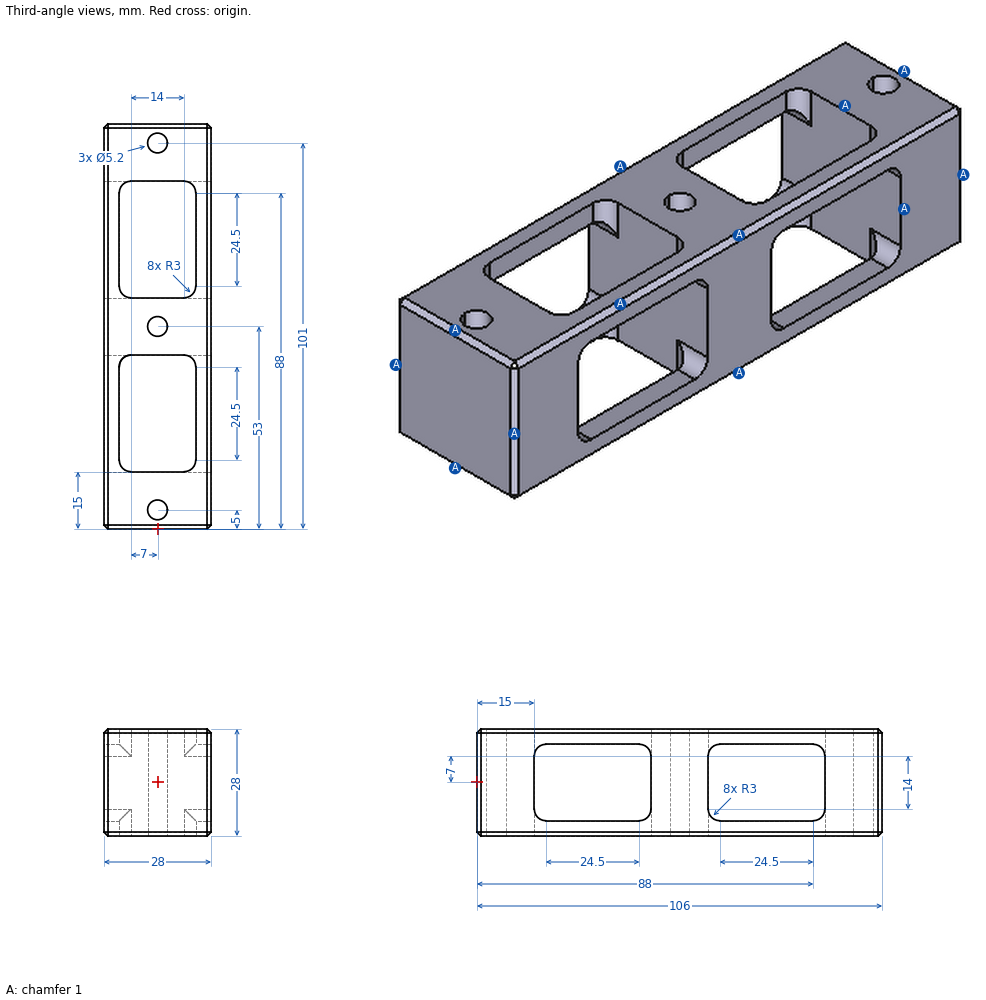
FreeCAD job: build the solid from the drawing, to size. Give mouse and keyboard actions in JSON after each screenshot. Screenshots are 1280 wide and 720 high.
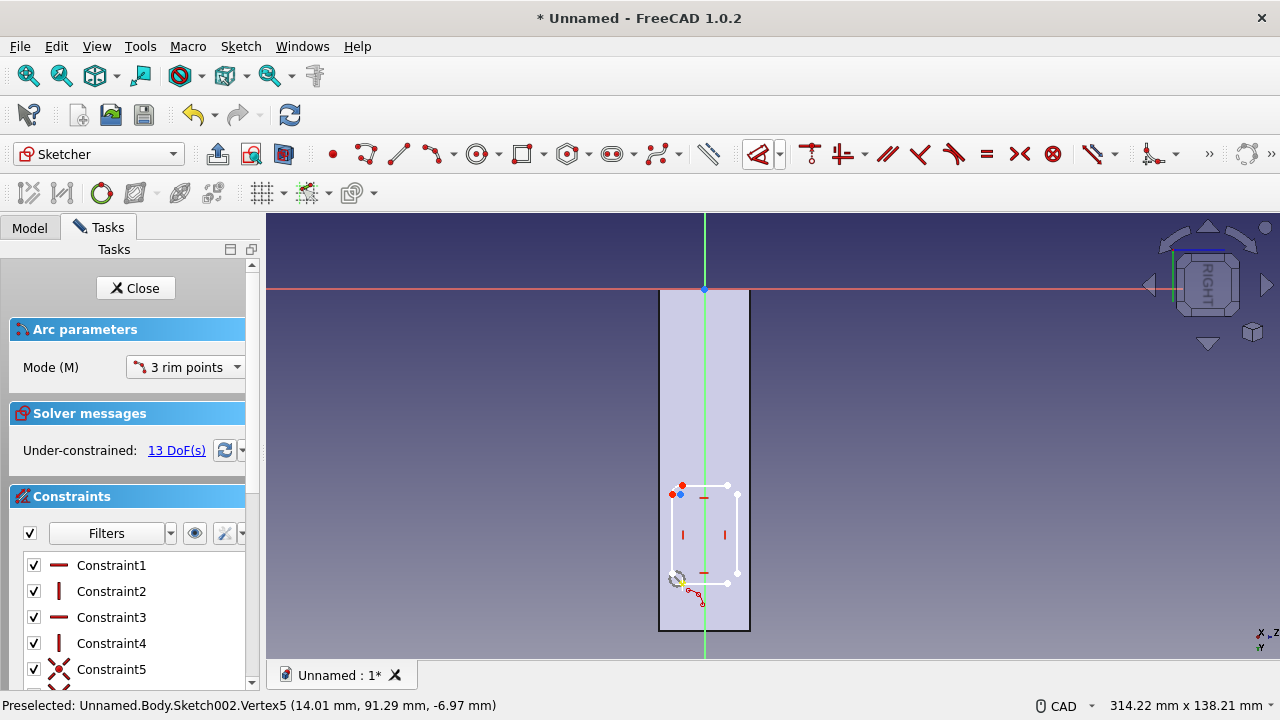
{"action": "scroll", "coordinate": [675, 580], "scroll_direction": "up", "scroll_amount": 9}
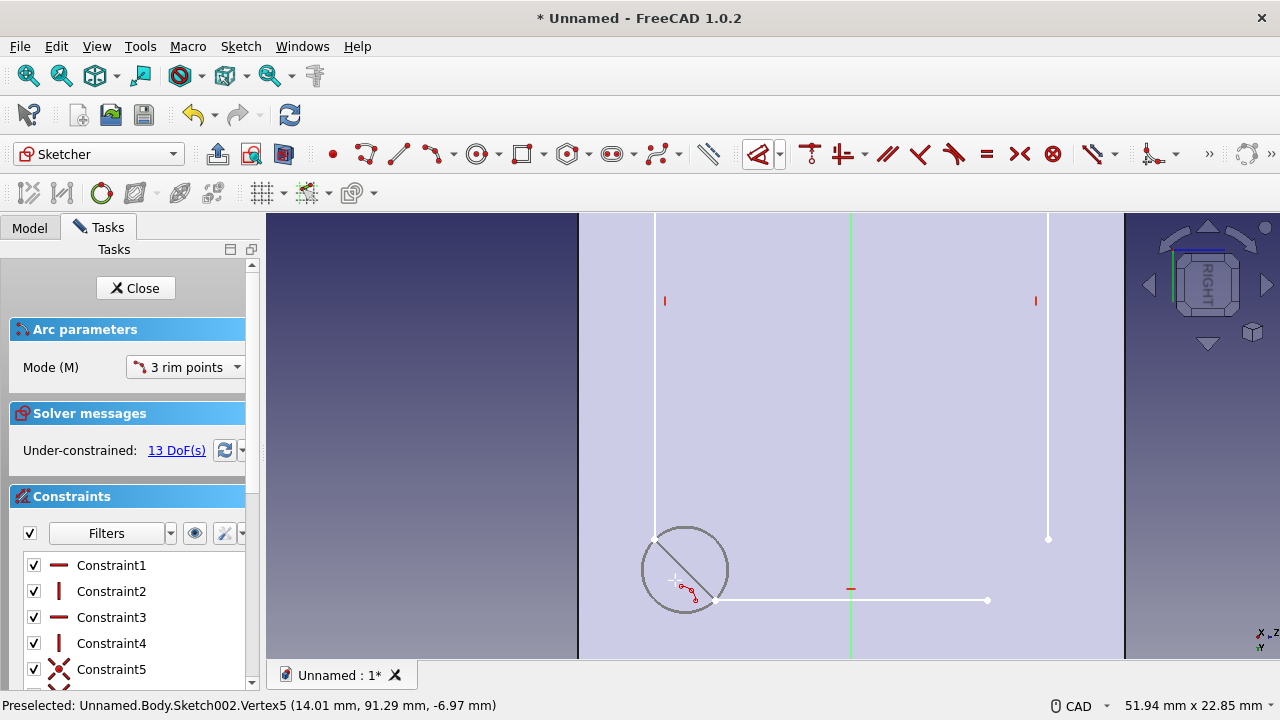
{"action": "left_click", "coordinate": [673, 577]}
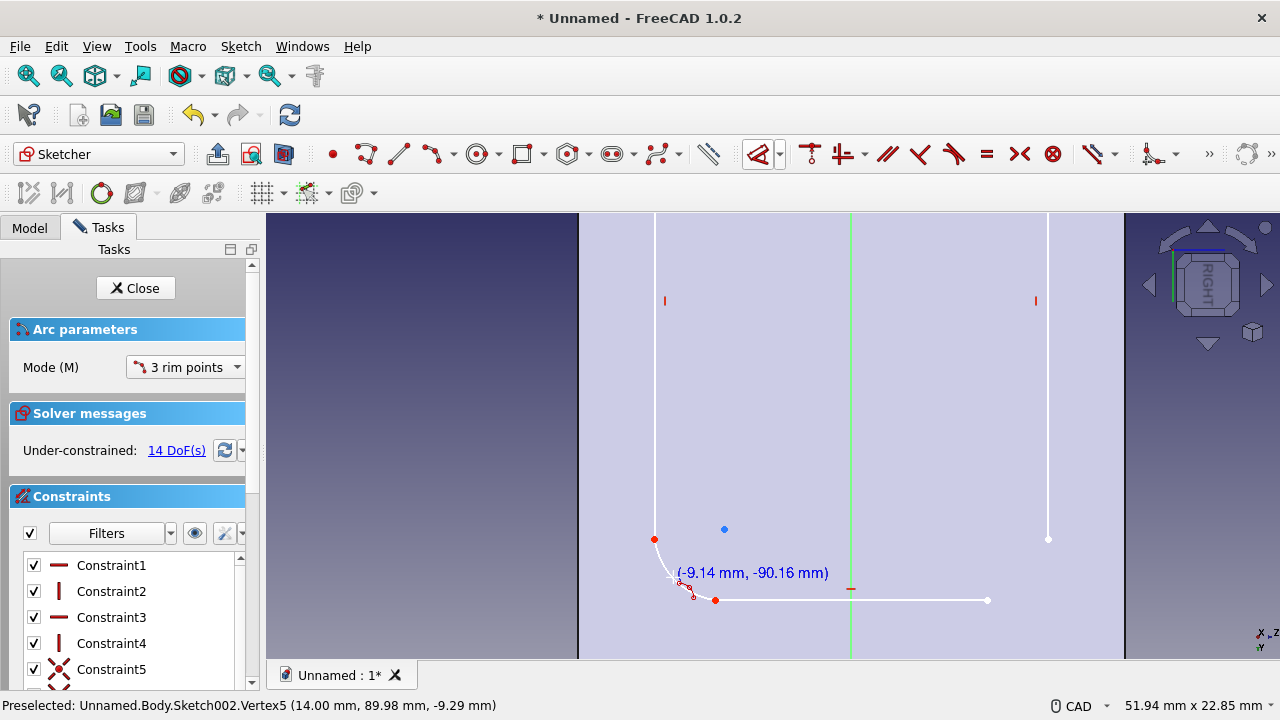
{"action": "scroll", "coordinate": [675, 581], "scroll_direction": "down", "scroll_amount": 9}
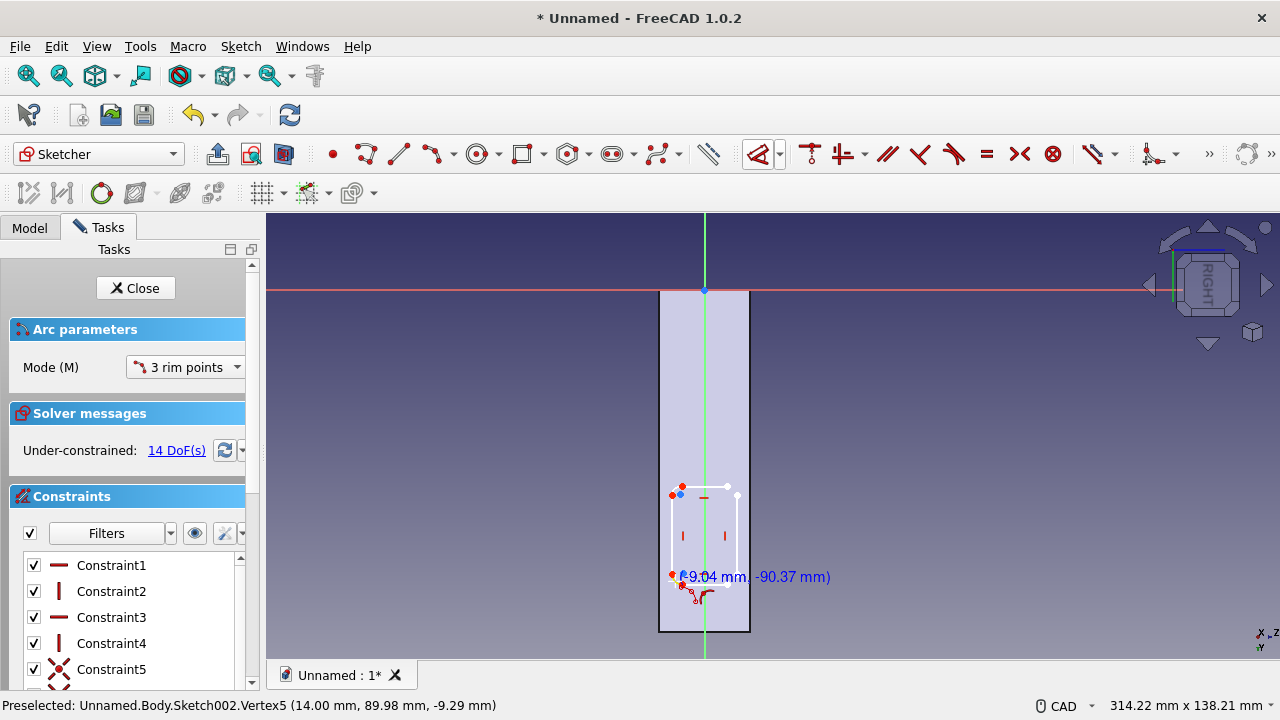
{"action": "left_click", "coordinate": [727, 585]}
{"action": "left_click", "coordinate": [737, 575]}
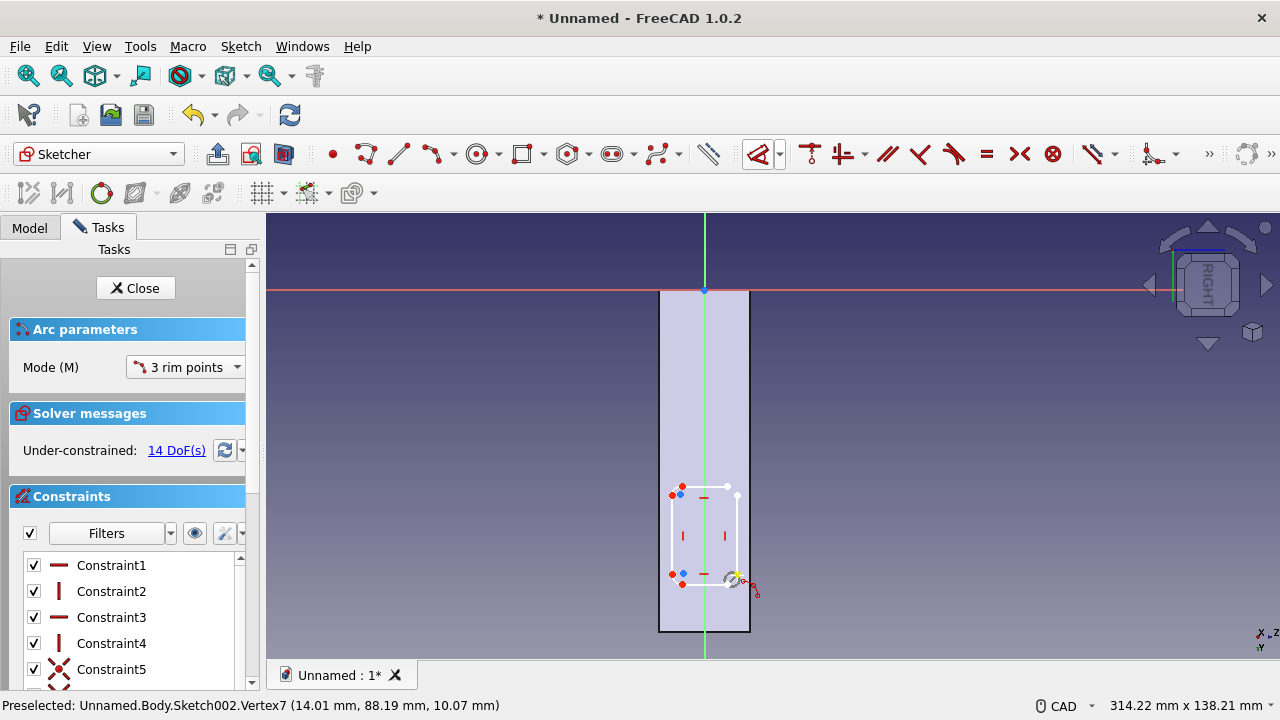
{"action": "scroll", "coordinate": [734, 581], "scroll_direction": "up", "scroll_amount": 9}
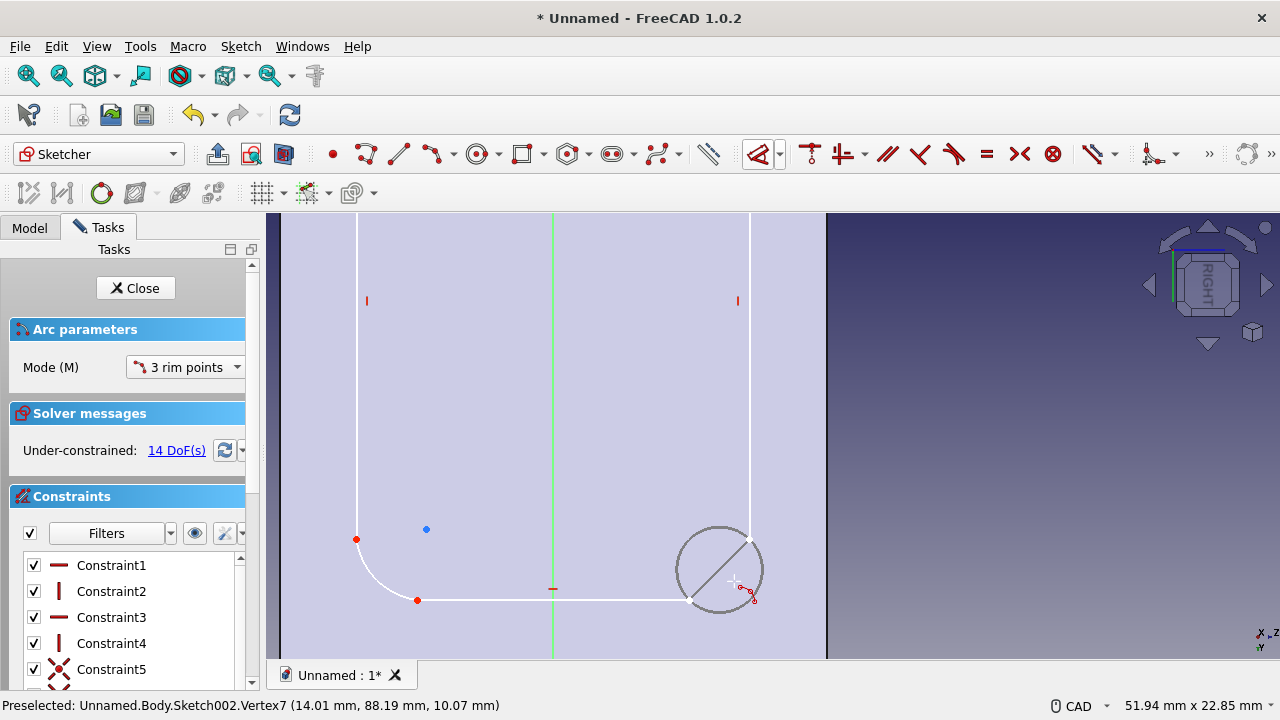
{"action": "left_click", "coordinate": [731, 577]}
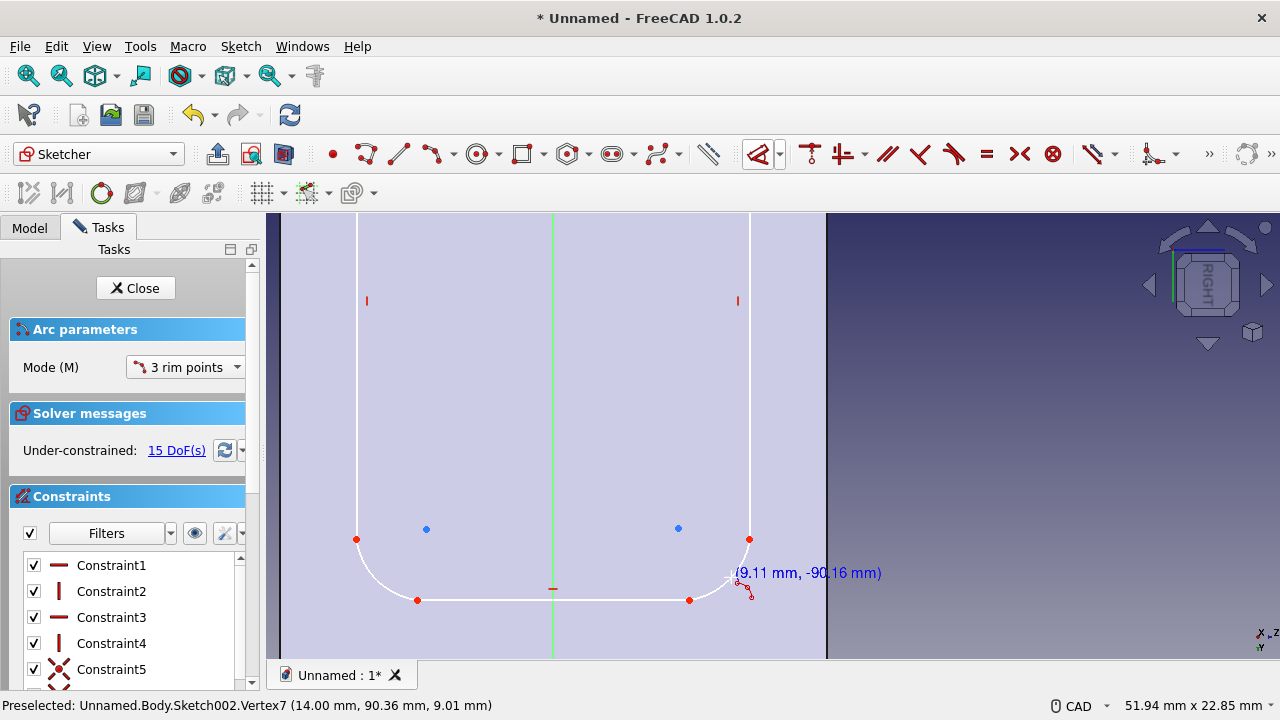
{"action": "scroll", "coordinate": [734, 581], "scroll_direction": "down", "scroll_amount": 9}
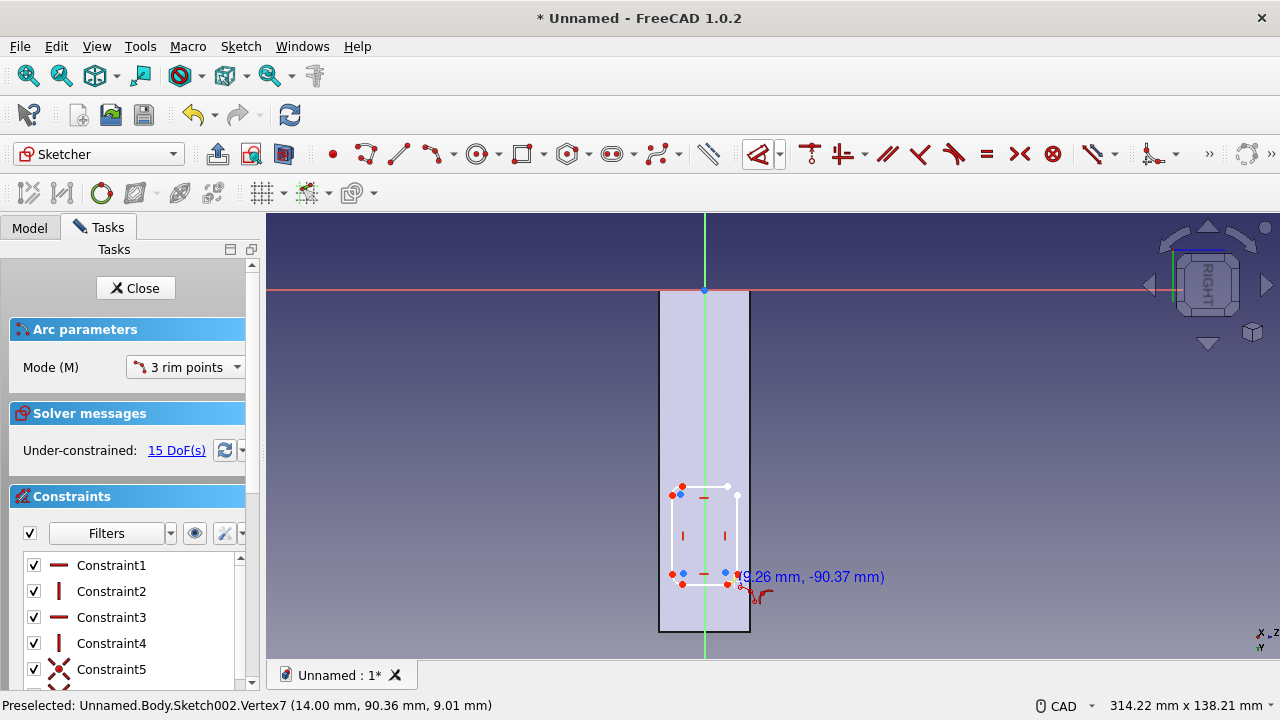
{"action": "left_click", "coordinate": [737, 496]}
{"action": "left_click", "coordinate": [727, 487]}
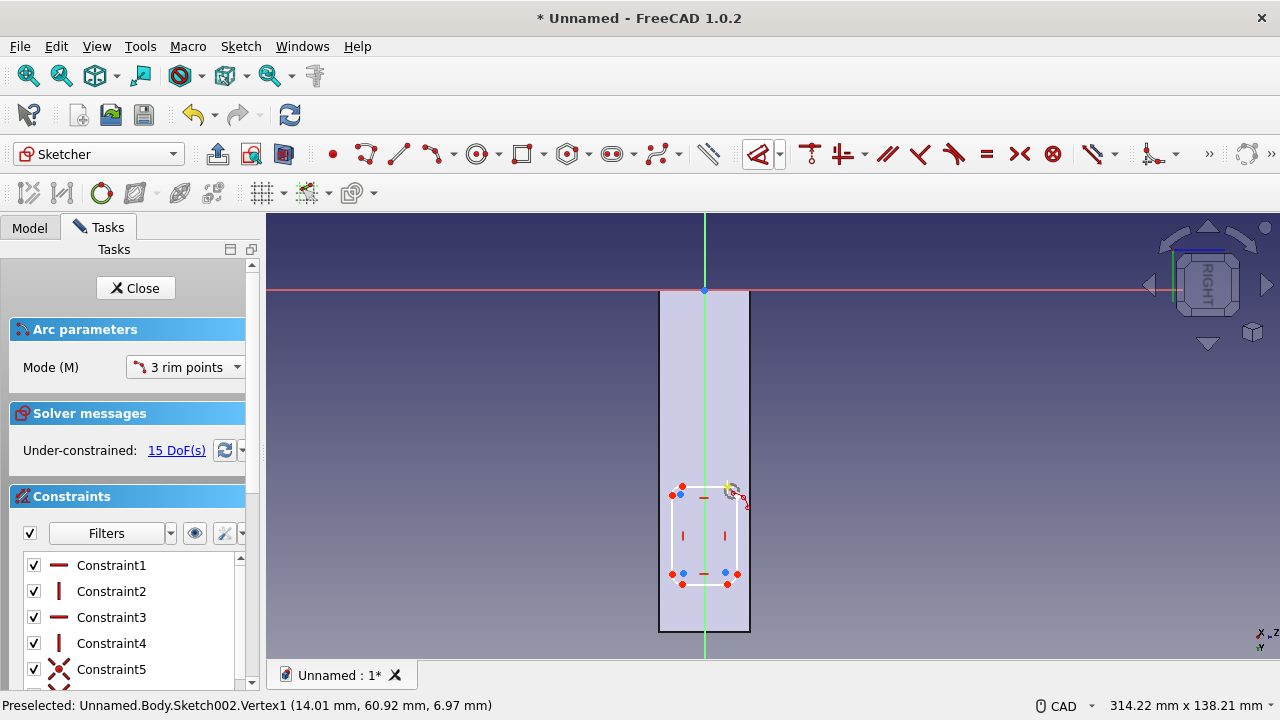
{"action": "scroll", "coordinate": [734, 488], "scroll_direction": "up", "scroll_amount": 9}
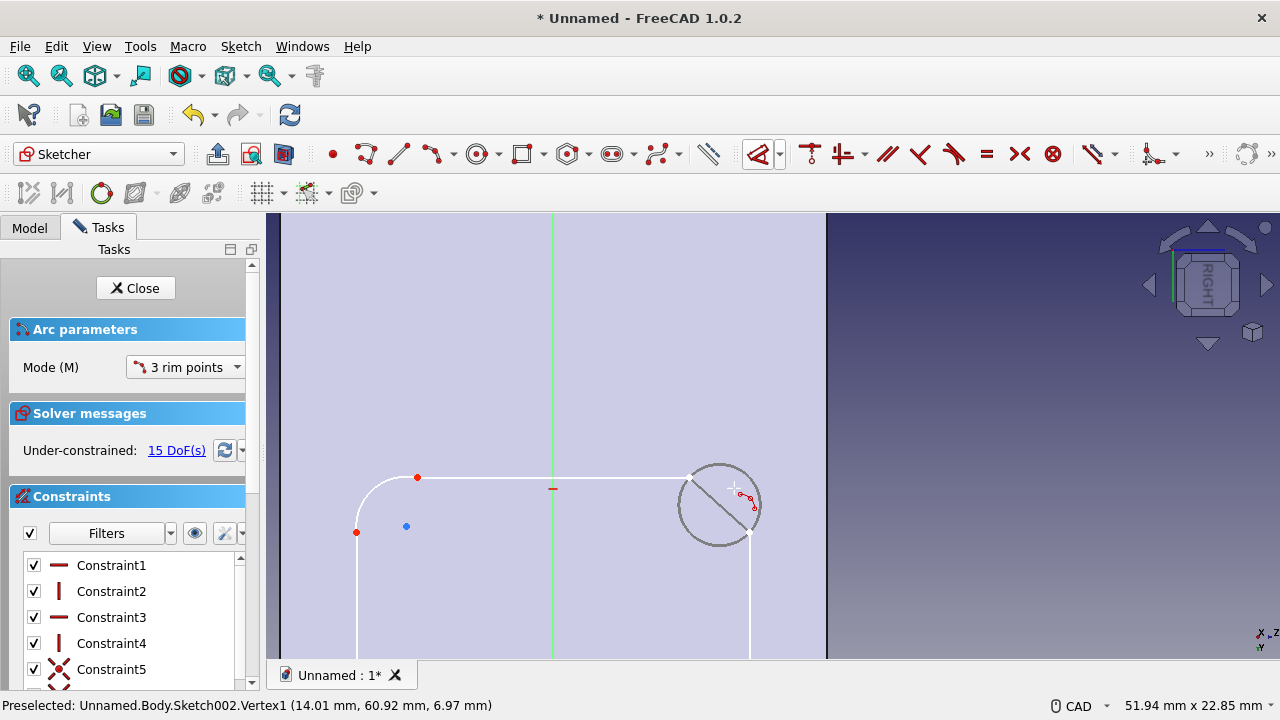
{"action": "left_click", "coordinate": [731, 487]}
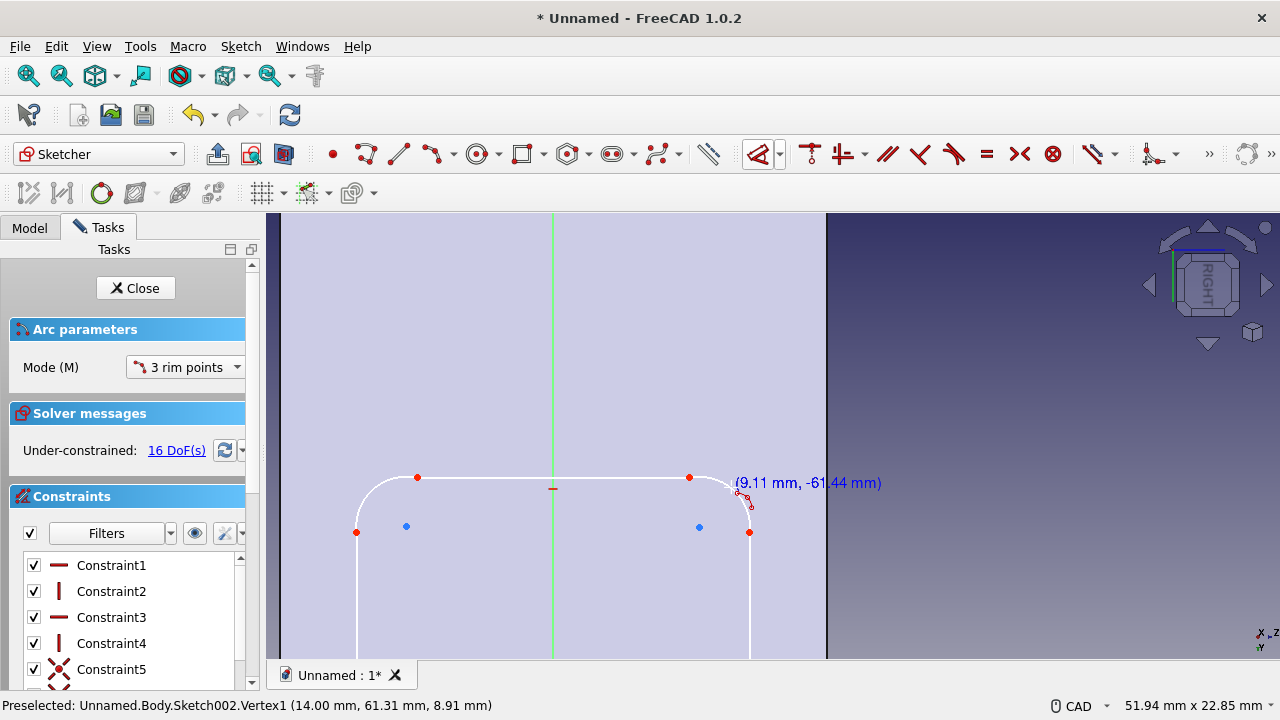
{"action": "left_click", "coordinate": [399, 154]}